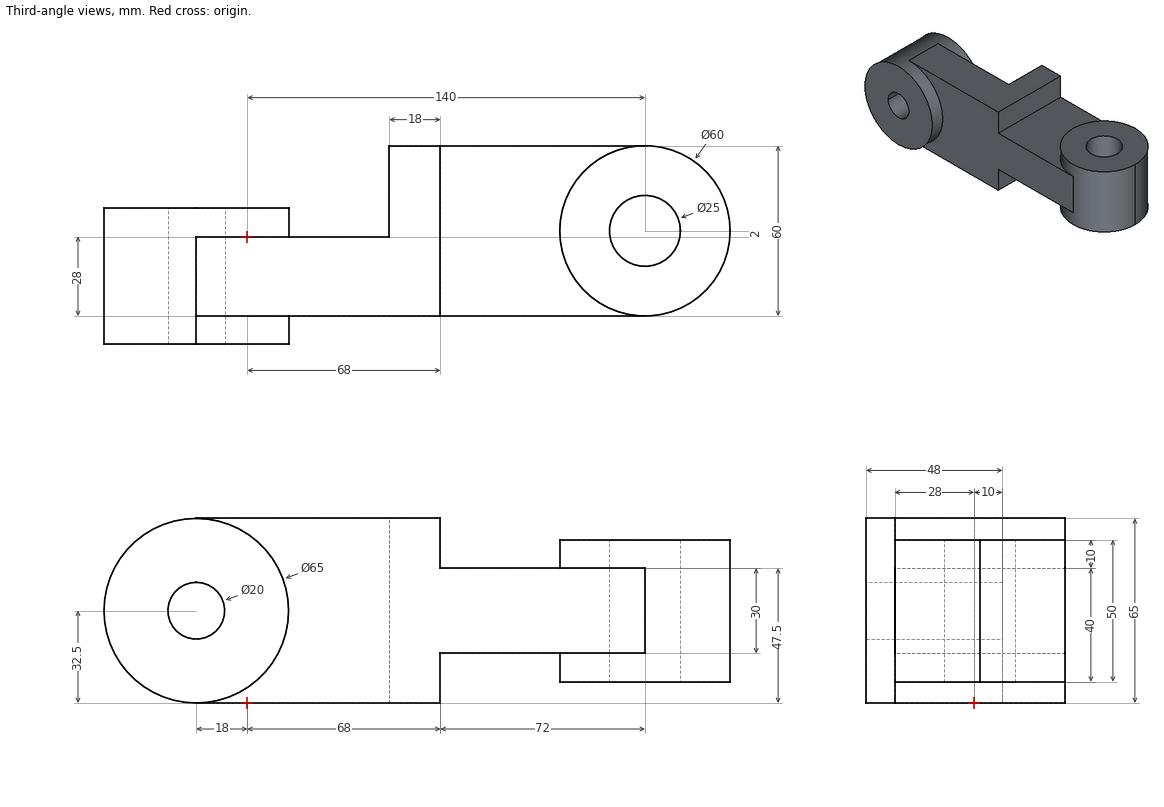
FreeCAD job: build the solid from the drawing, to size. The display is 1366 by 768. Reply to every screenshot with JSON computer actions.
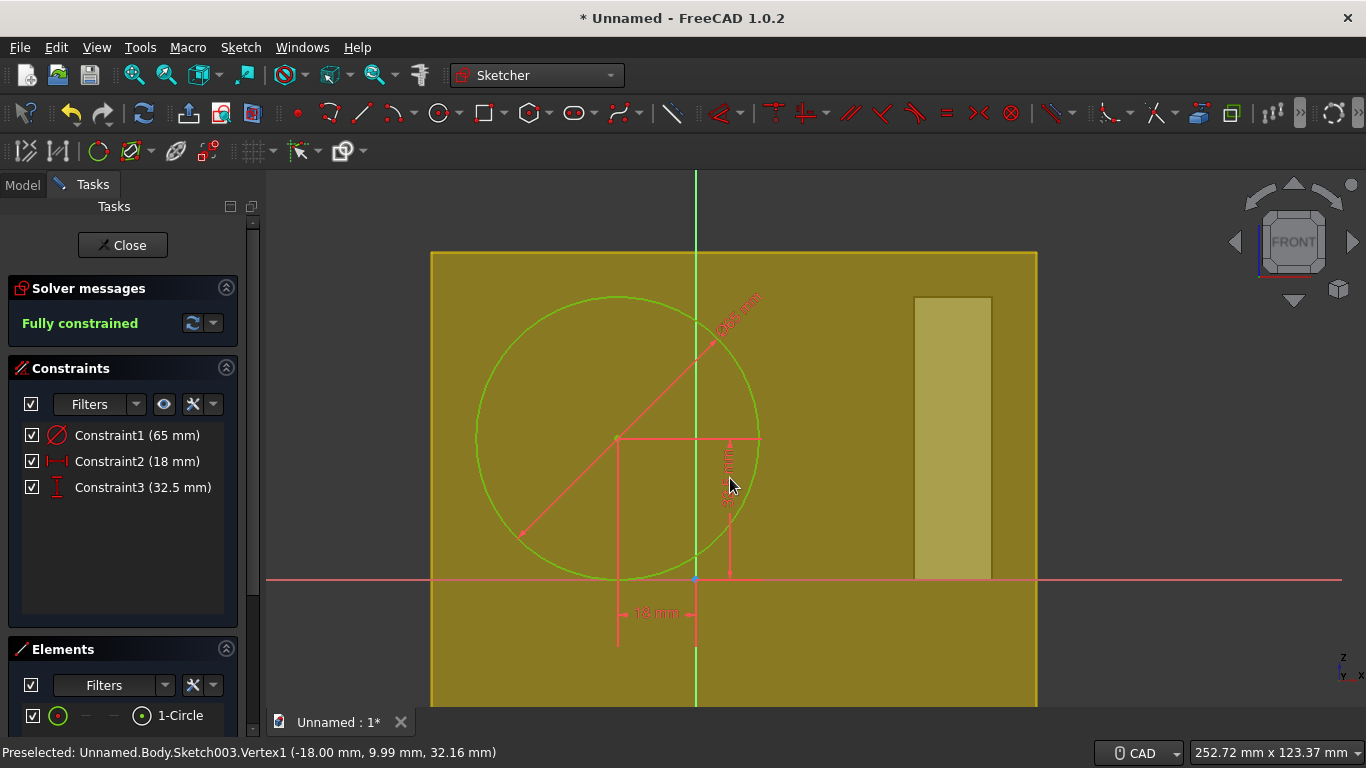
{"action": "left_click", "coordinate": [123, 245]}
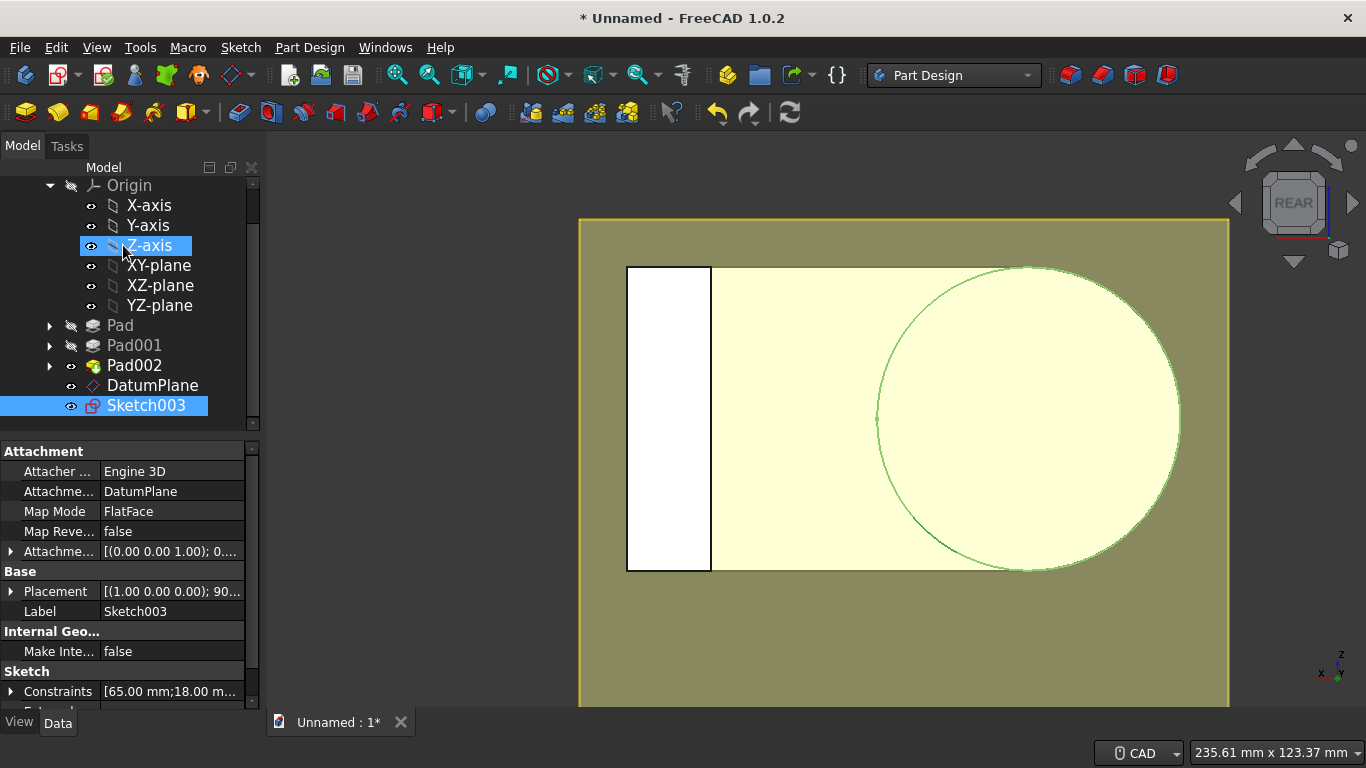
{"action": "left_click", "coordinate": [26, 112]}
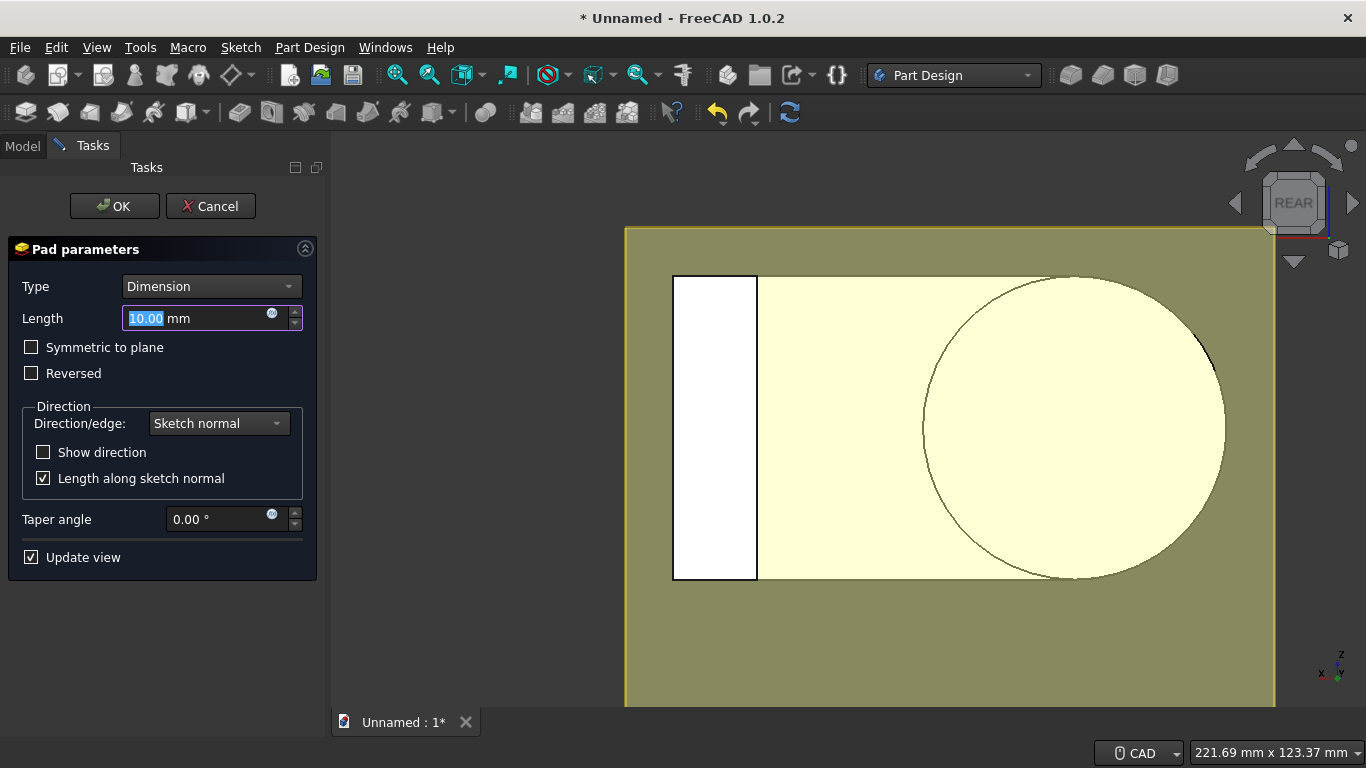
{"action": "type", "text": "10"}
{"action": "key", "text": "Tab"}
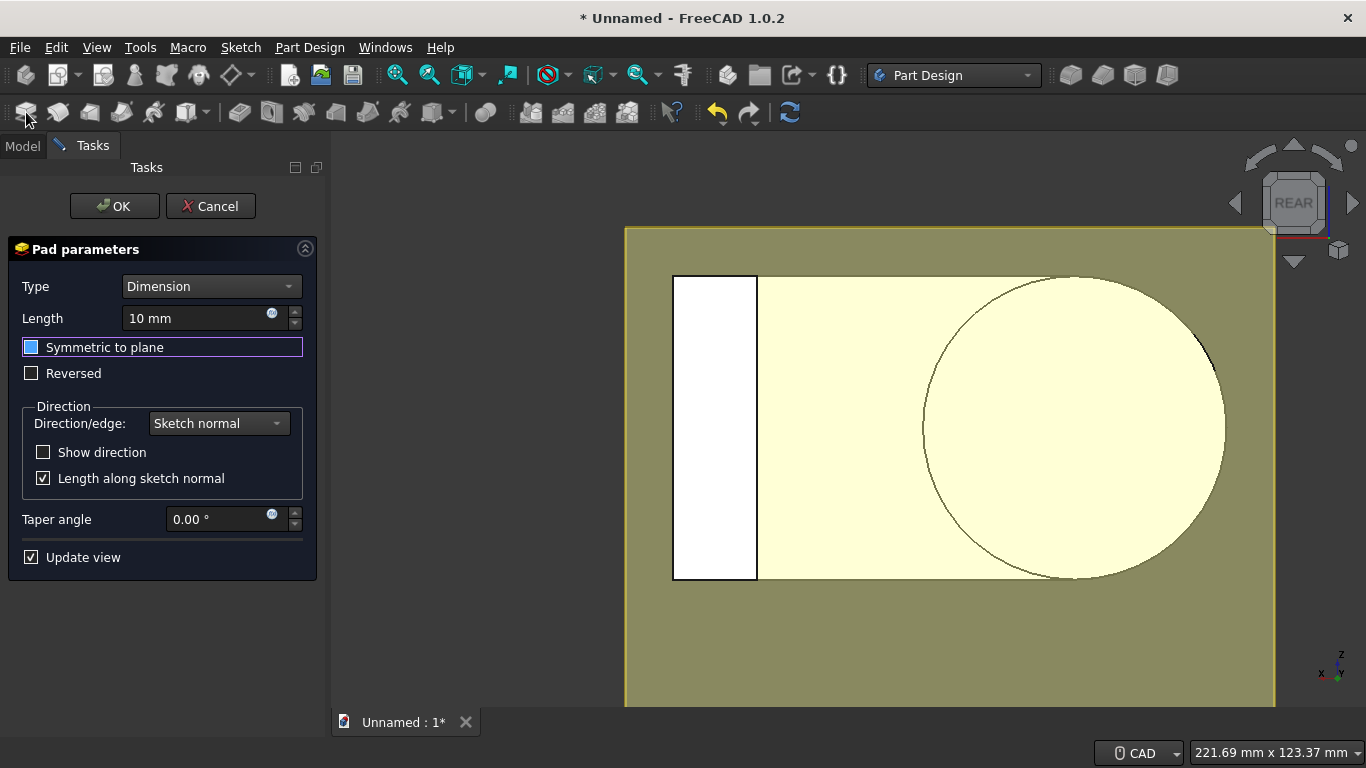
{"action": "left_click", "coordinate": [115, 206]}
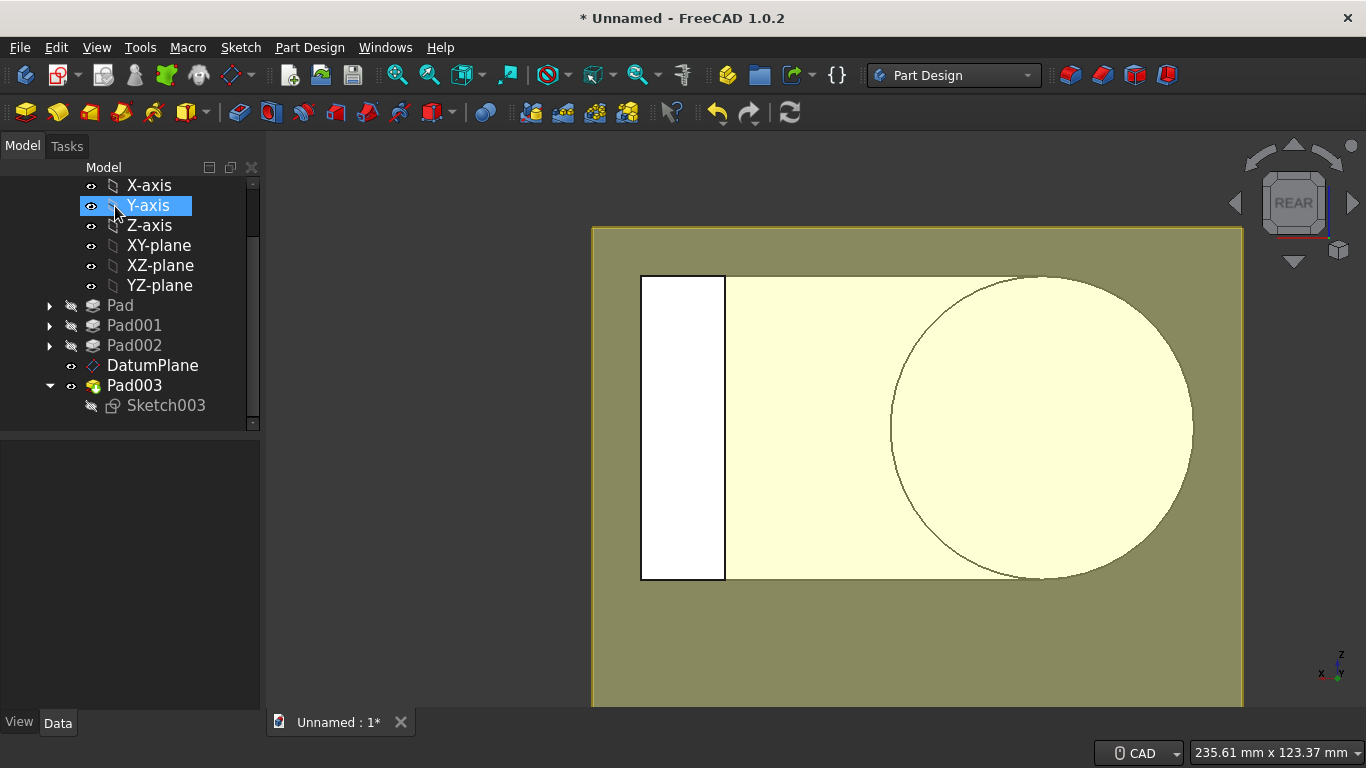
{"action": "left_click", "coordinate": [116, 366]}
{"action": "key", "text": "space"}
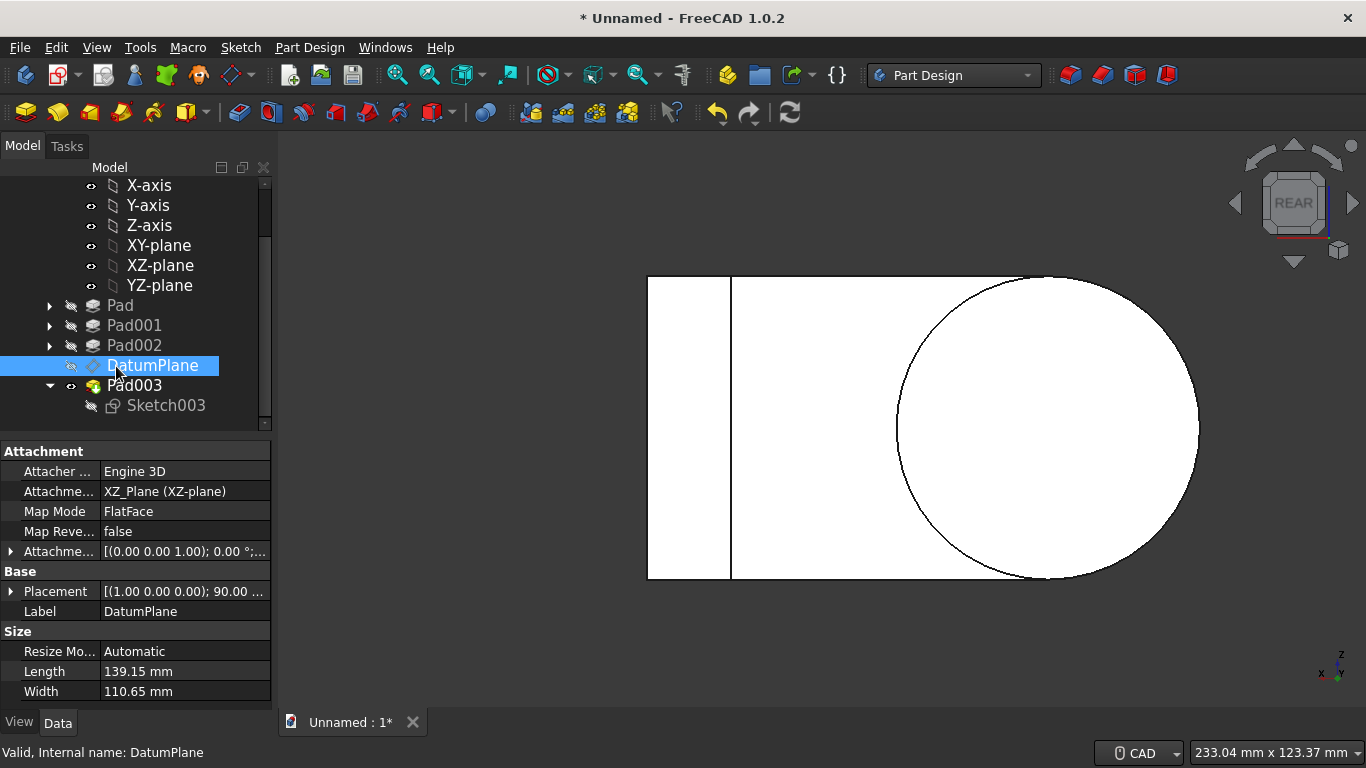
{"action": "scroll", "coordinate": [160, 301], "scroll_direction": "down", "scroll_amount": 3}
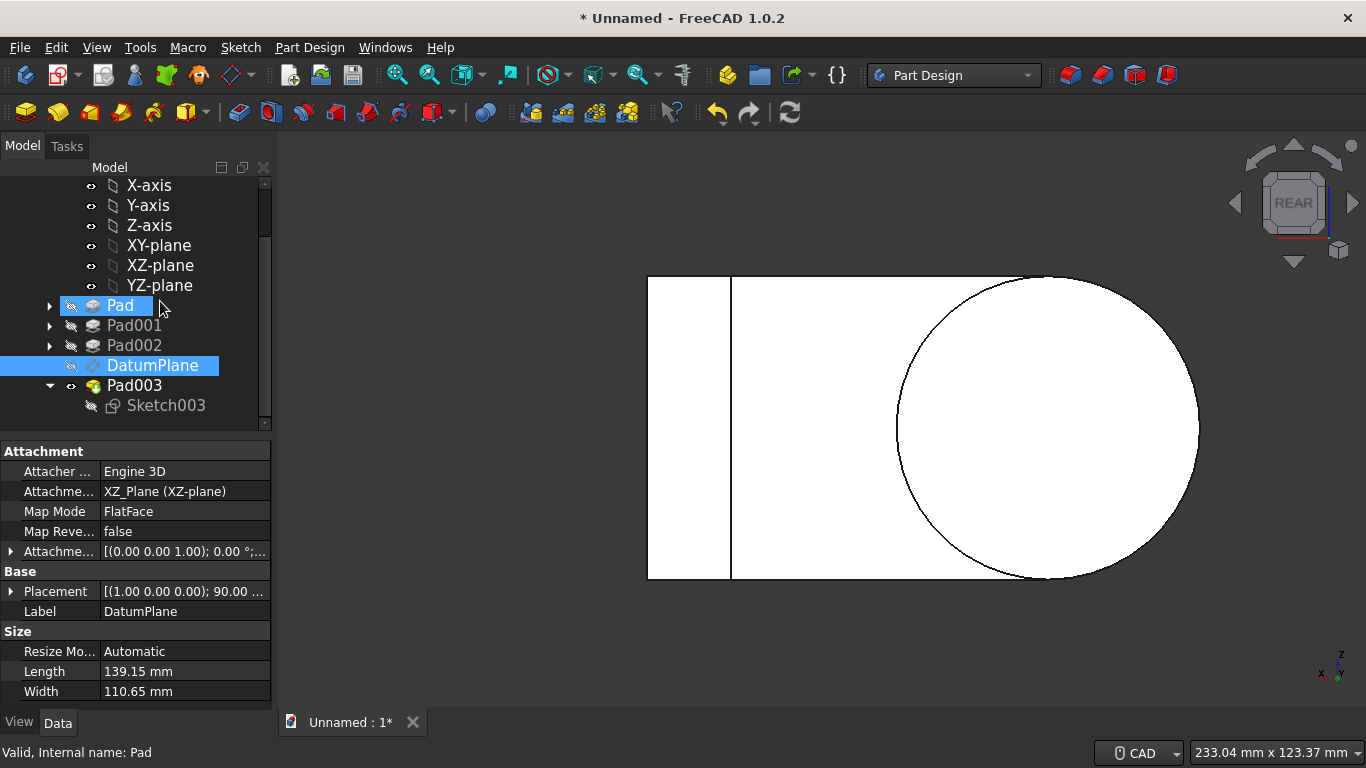
{"action": "scroll", "coordinate": [160, 301], "scroll_direction": "up", "scroll_amount": 15}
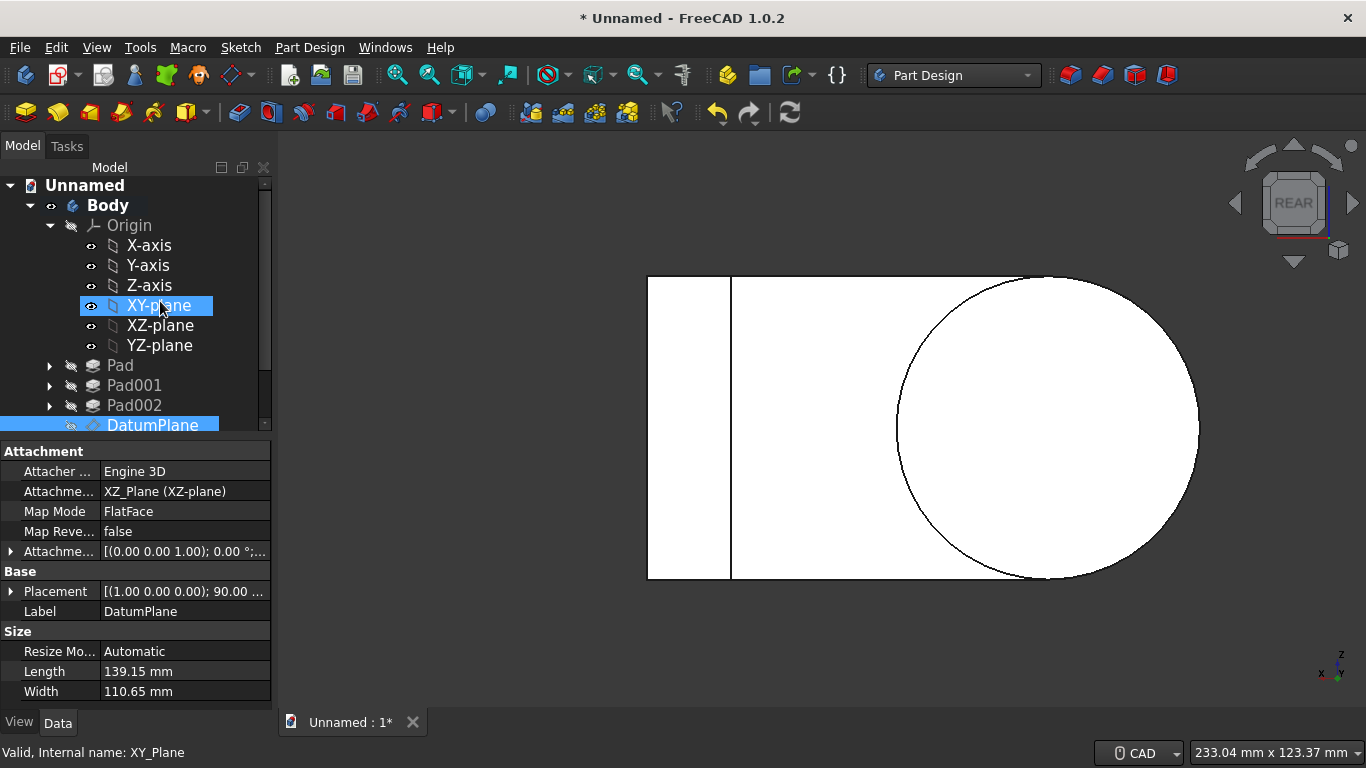
{"action": "left_click", "coordinate": [136, 326]}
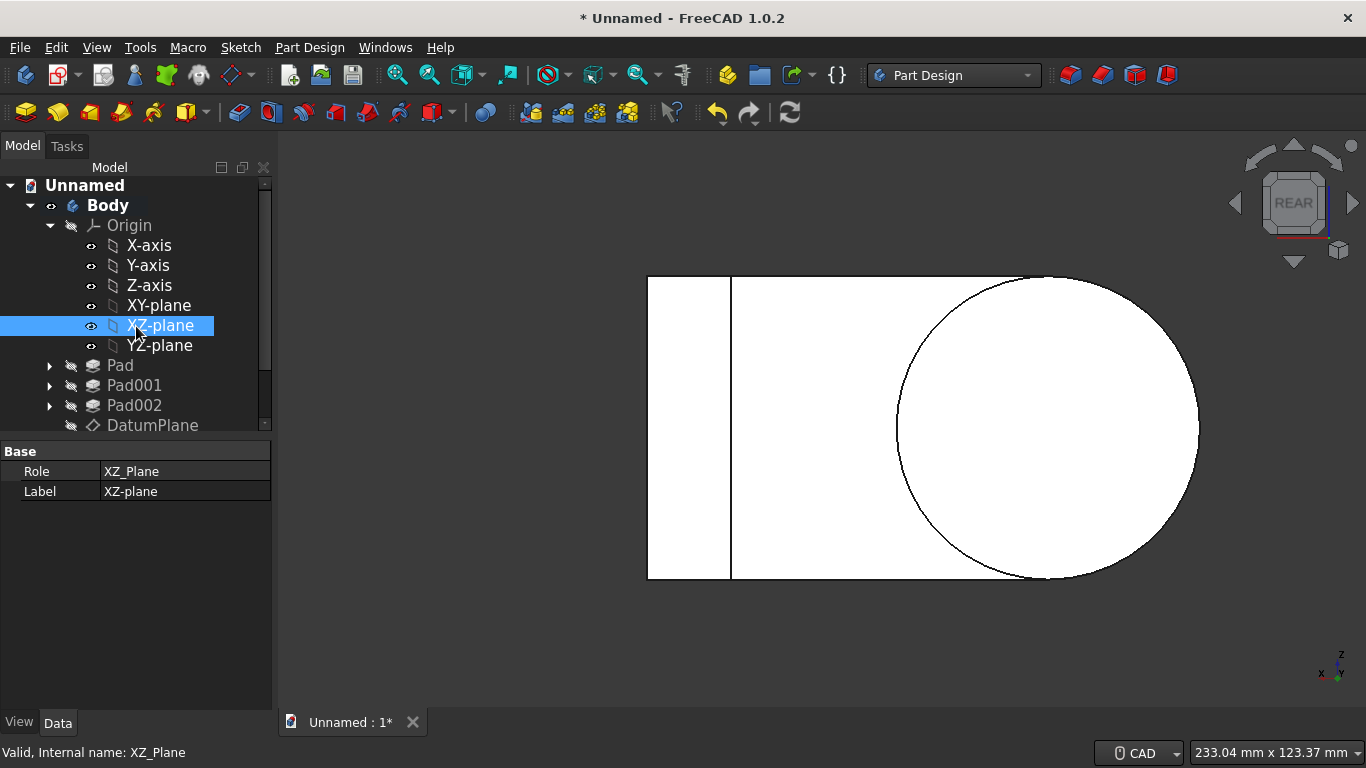
{"action": "left_click", "coordinate": [232, 76]}